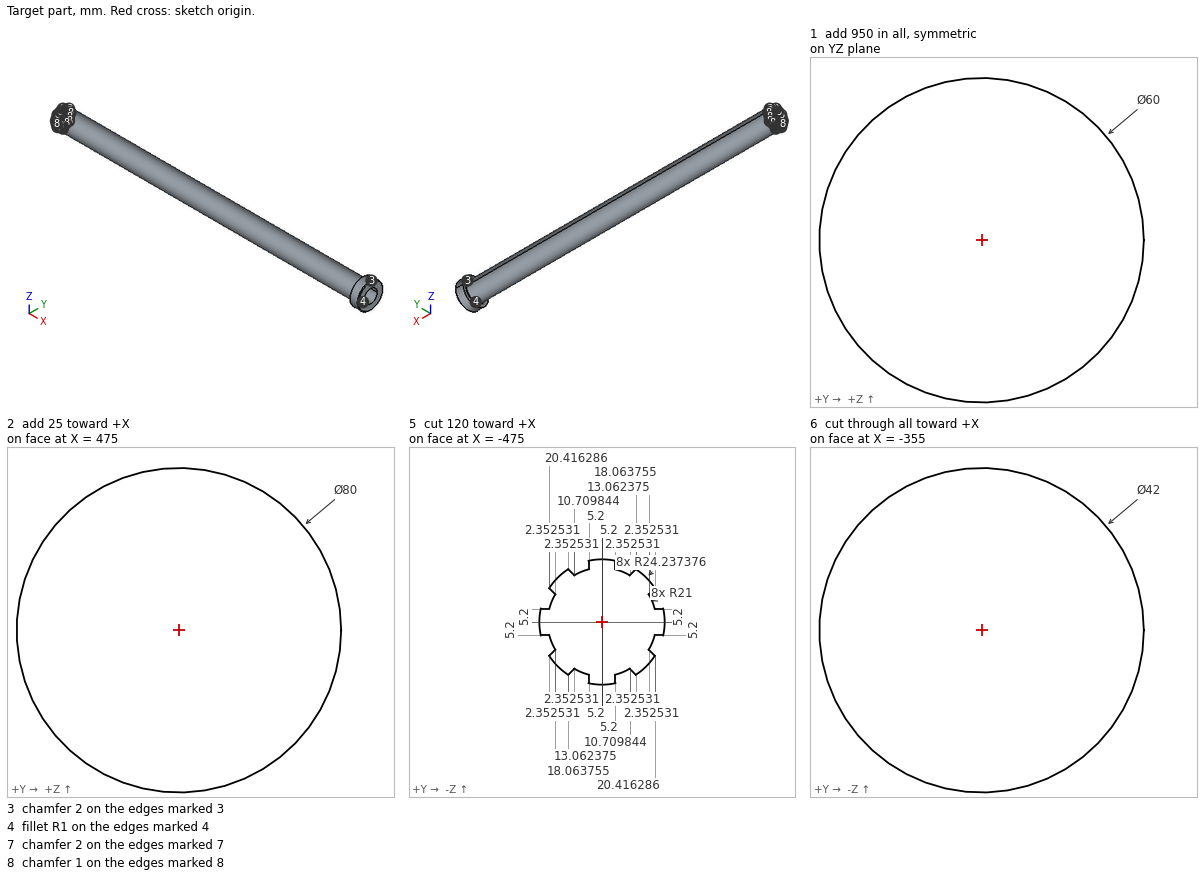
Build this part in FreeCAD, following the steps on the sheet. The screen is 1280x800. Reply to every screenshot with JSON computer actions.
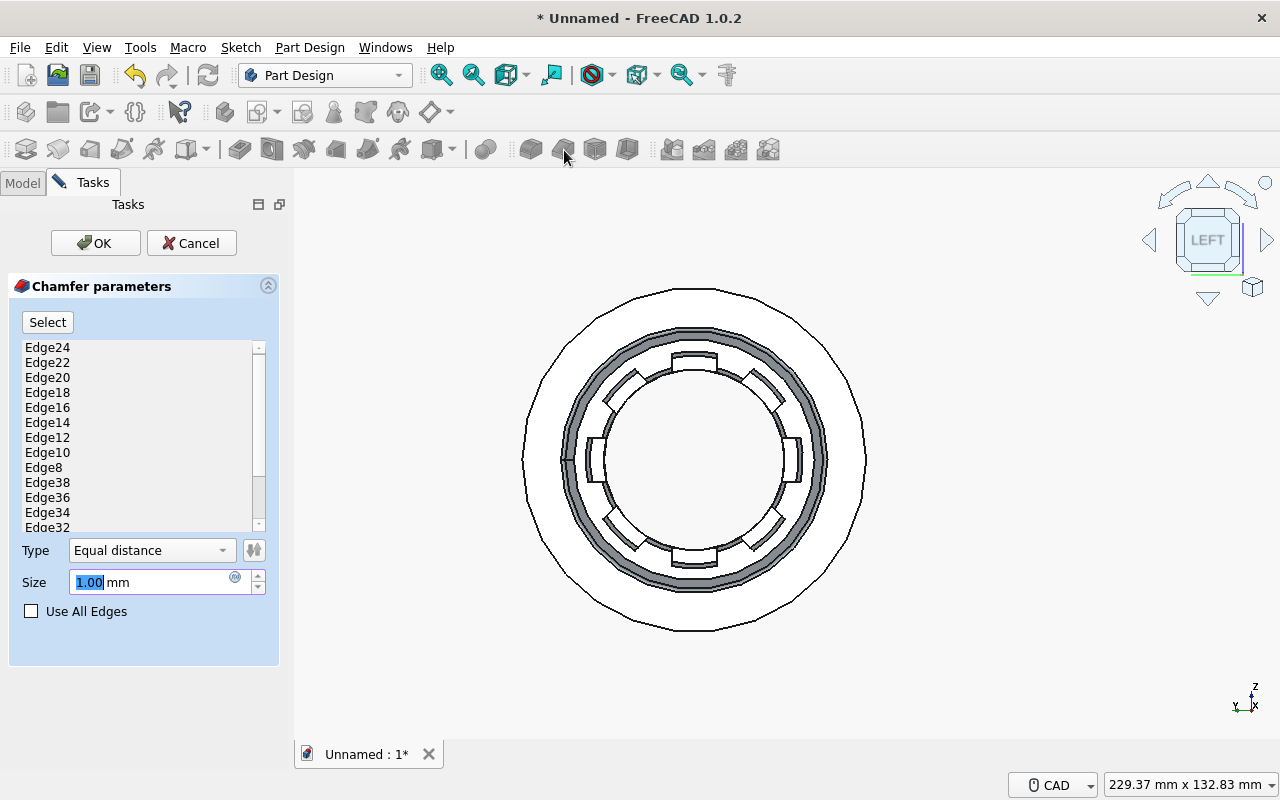
{"action": "type", "text": "1"}
{"action": "key", "text": "Tab"}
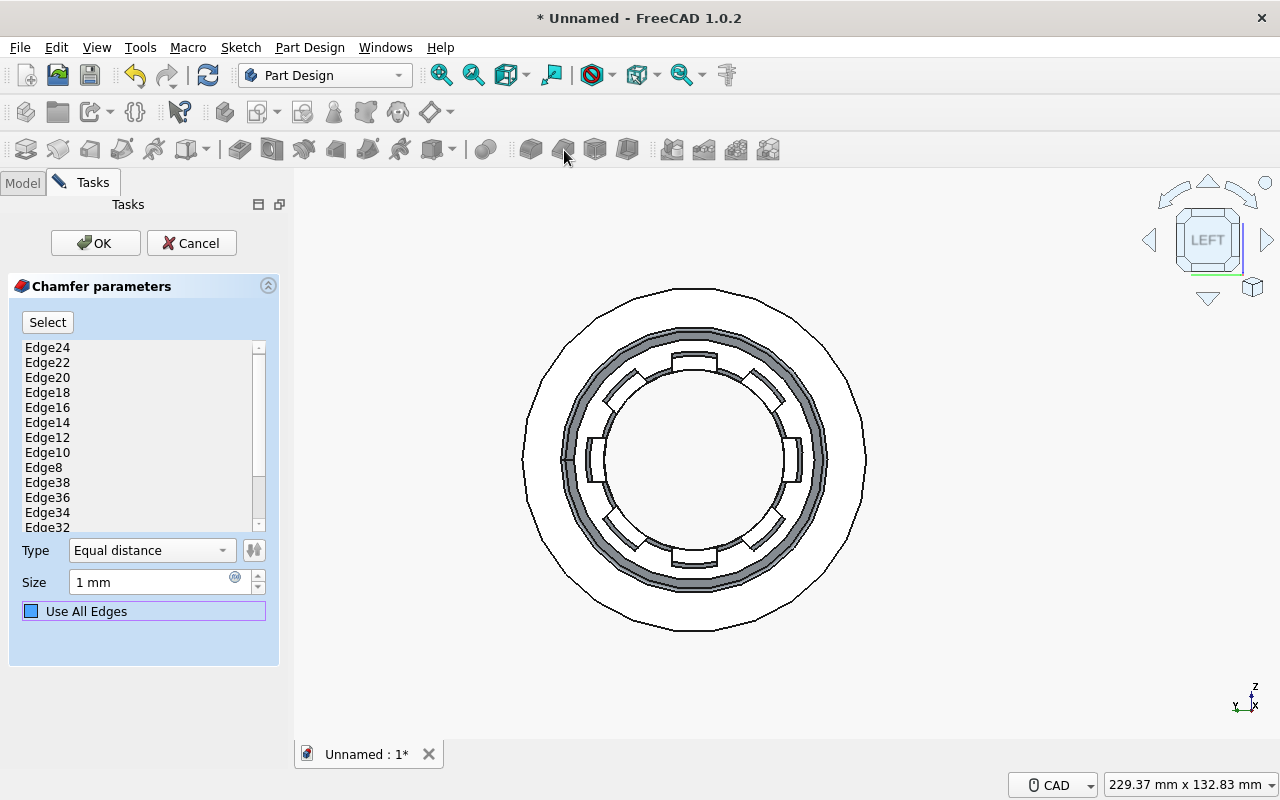
{"action": "left_click", "coordinate": [96, 243]}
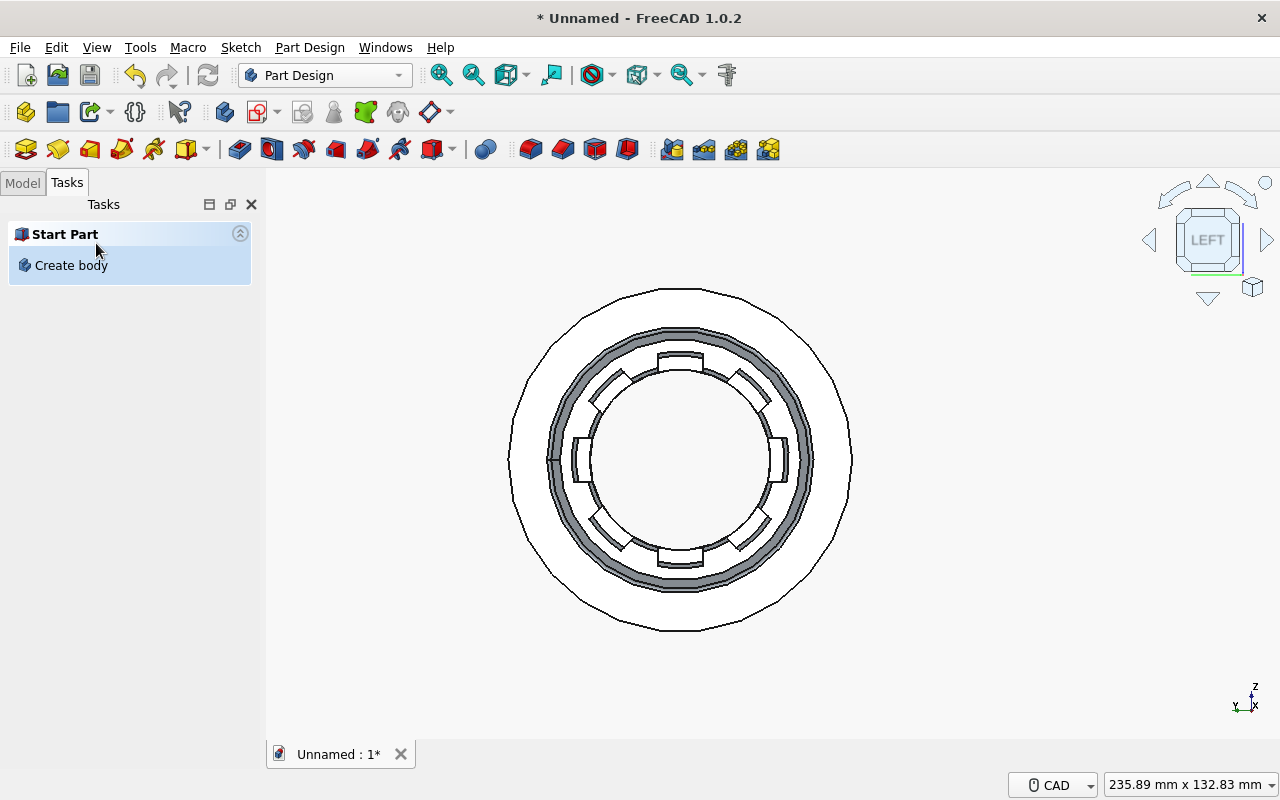
{"action": "key", "text": "0"}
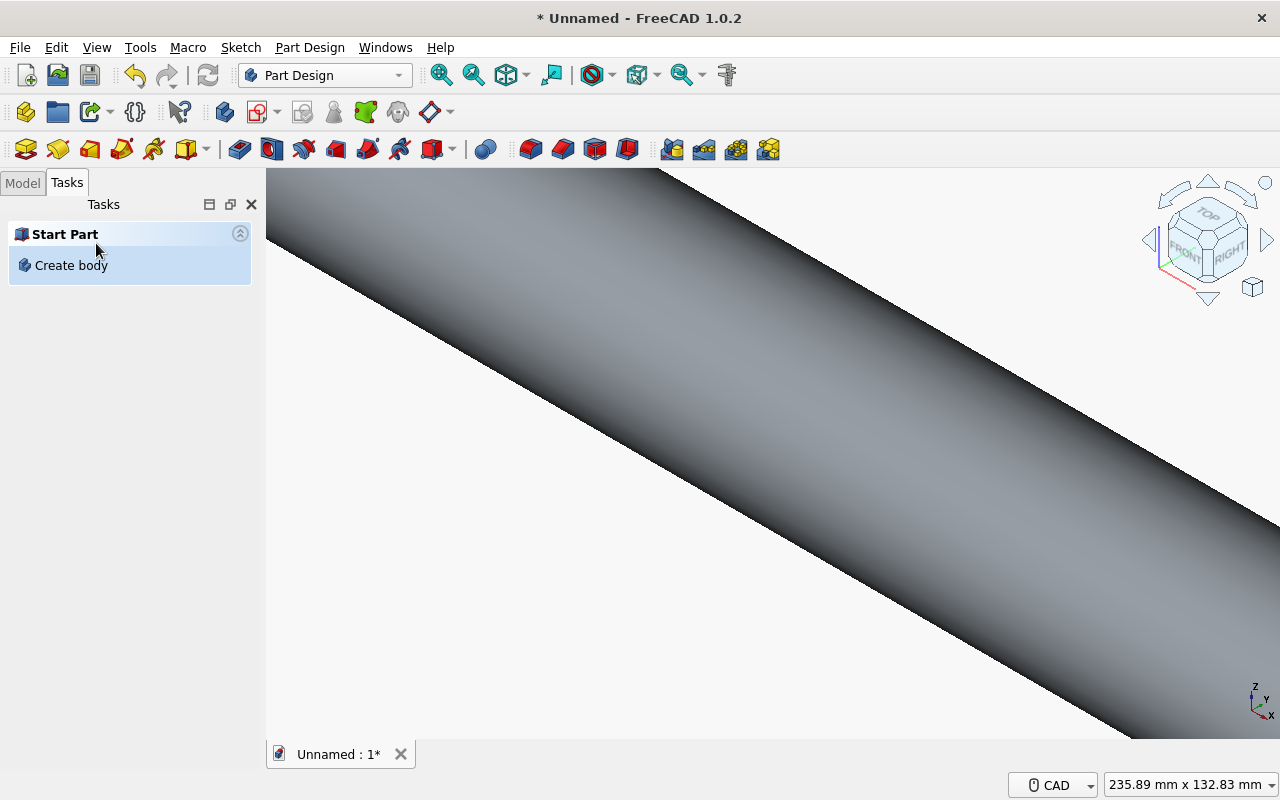
{"action": "left_click", "coordinate": [442, 76]}